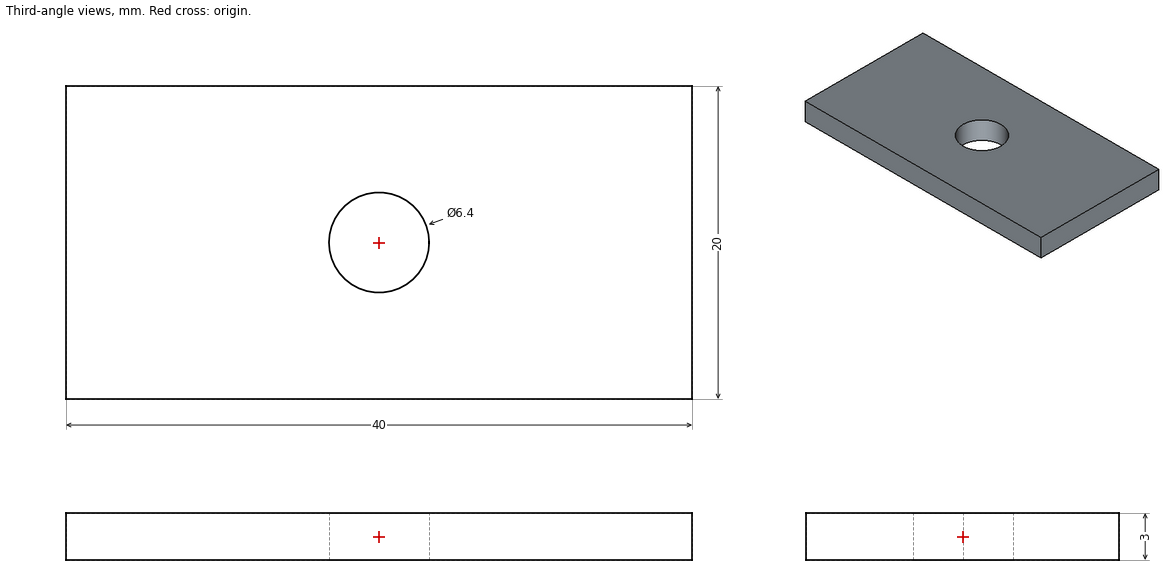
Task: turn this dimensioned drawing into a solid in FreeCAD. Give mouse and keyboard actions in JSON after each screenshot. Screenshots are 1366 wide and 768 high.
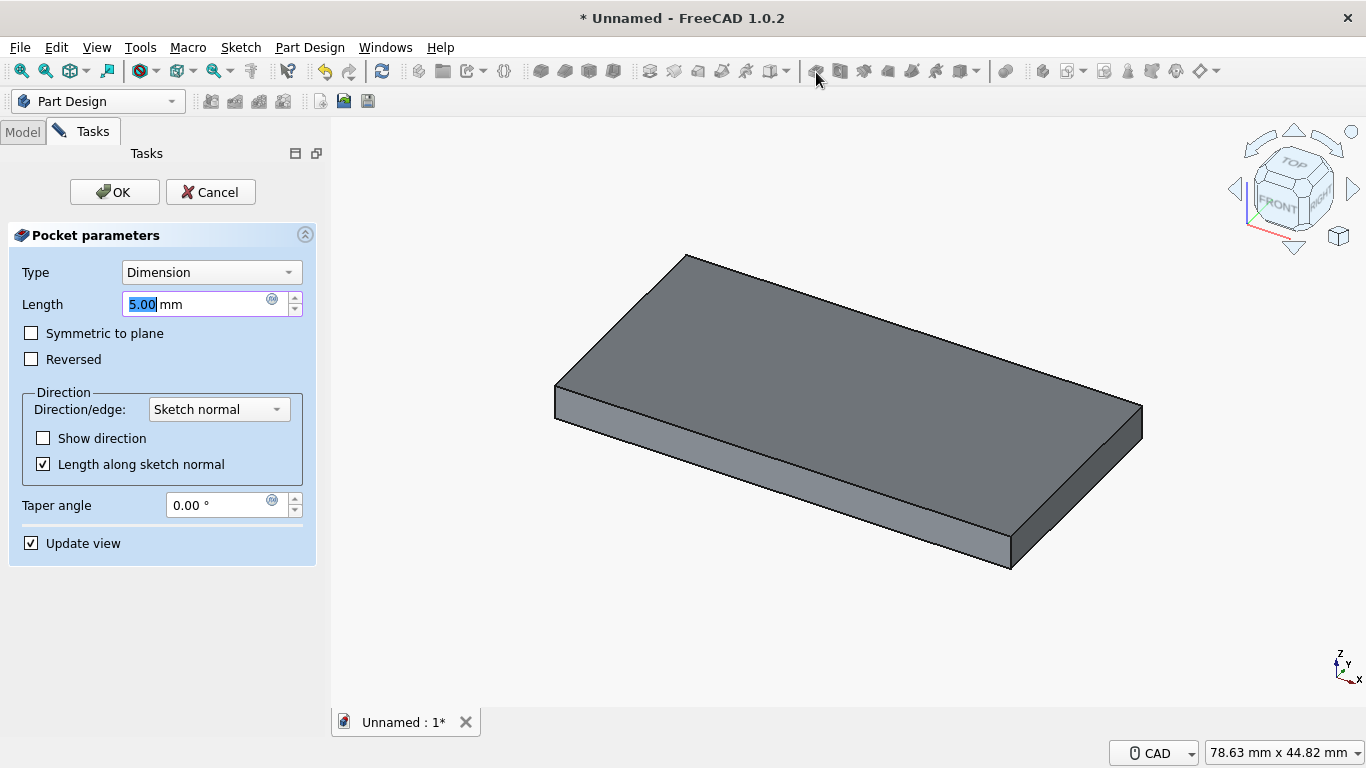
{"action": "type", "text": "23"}
{"action": "key", "text": "Tab"}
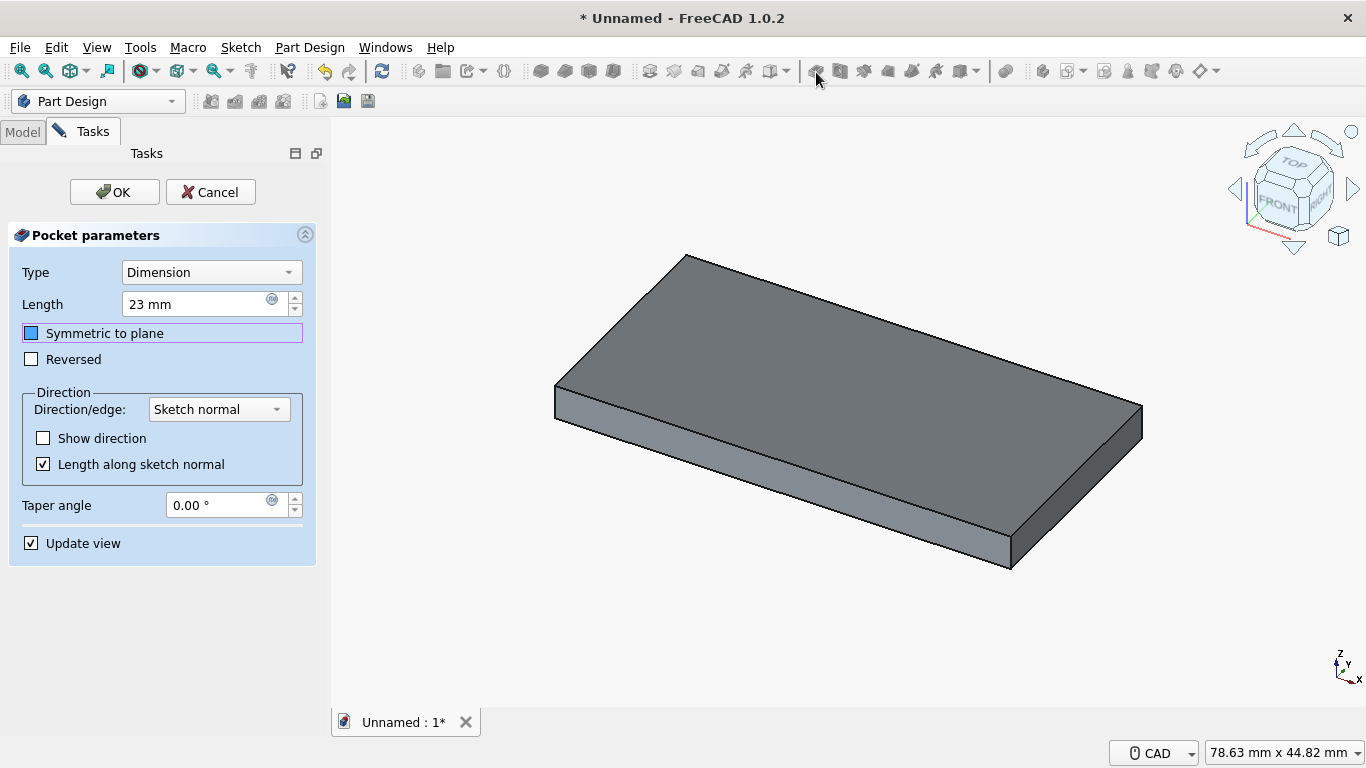
{"action": "left_click", "coordinate": [30, 333]}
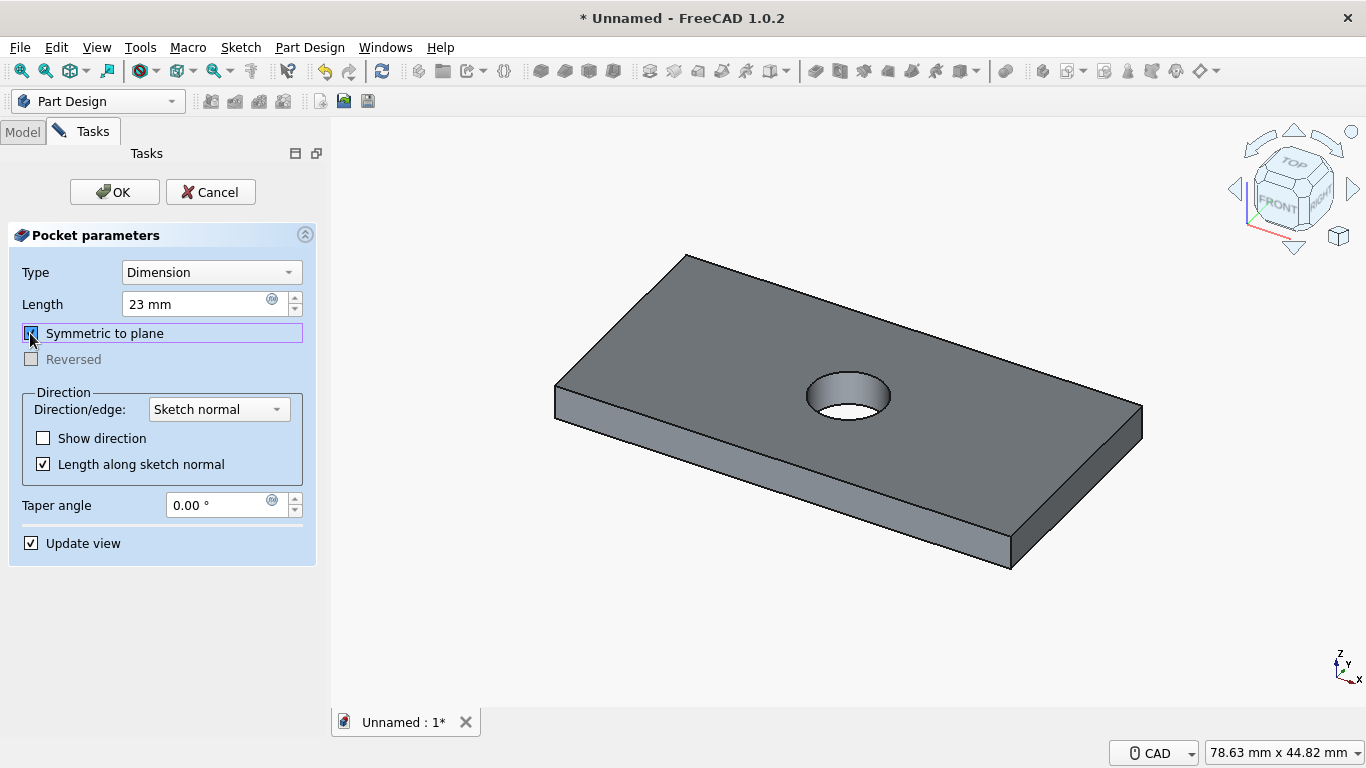
{"action": "left_click", "coordinate": [115, 192]}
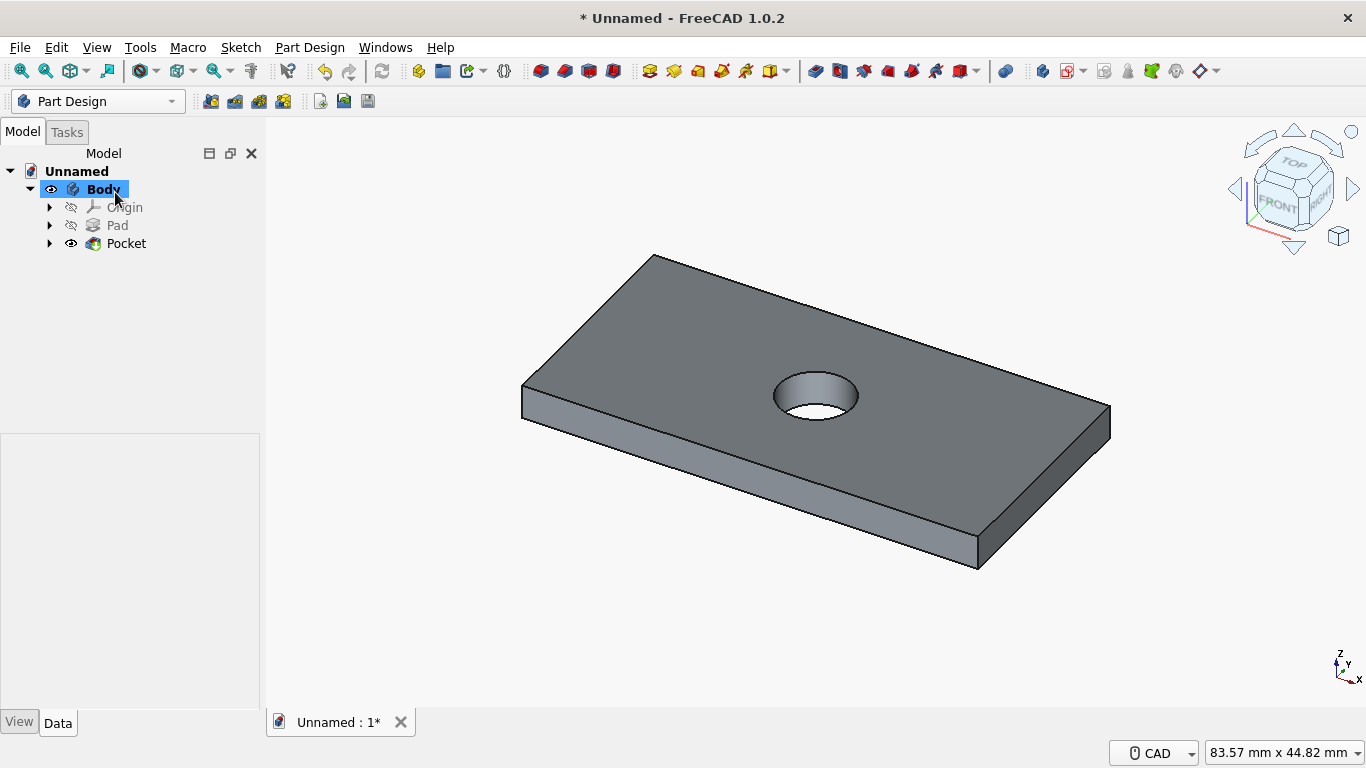
{"action": "key", "text": "0"}